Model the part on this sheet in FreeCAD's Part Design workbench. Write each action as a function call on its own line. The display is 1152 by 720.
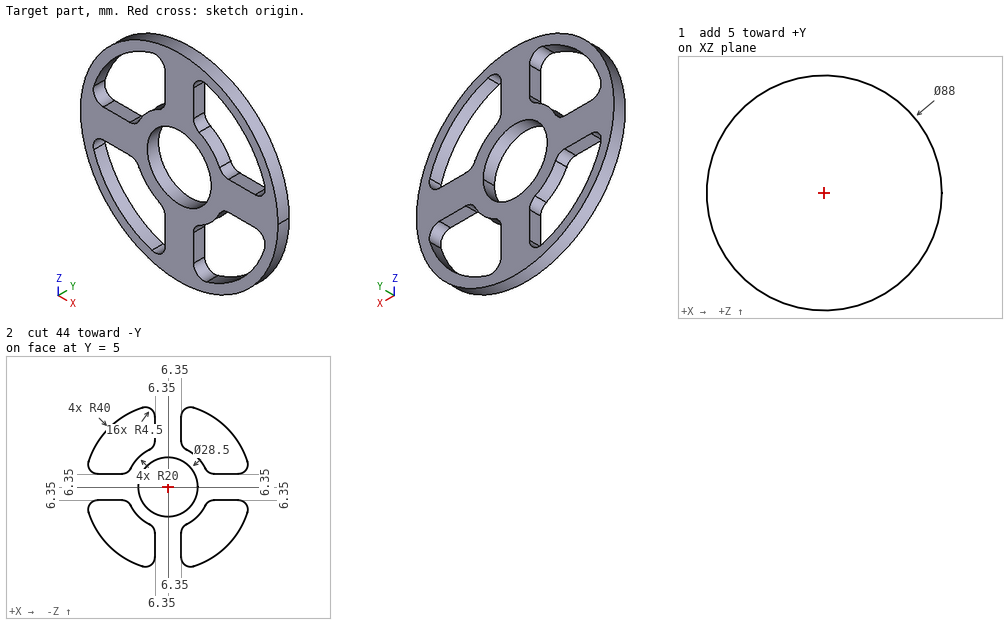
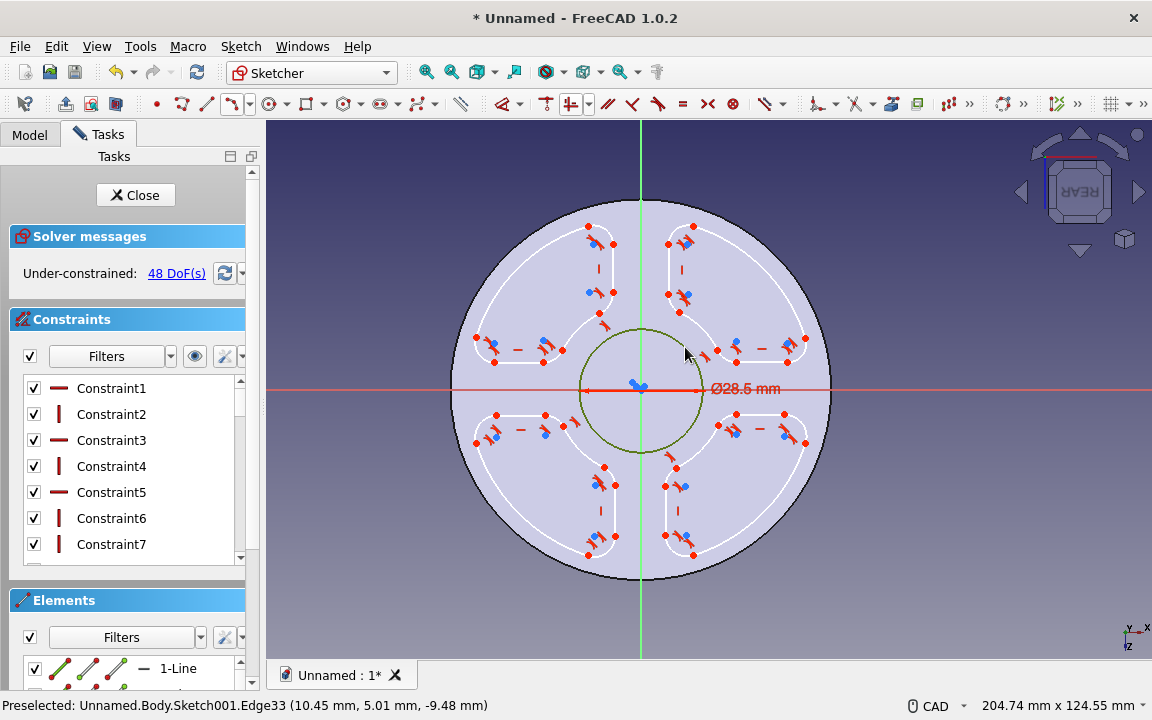
click(586, 322)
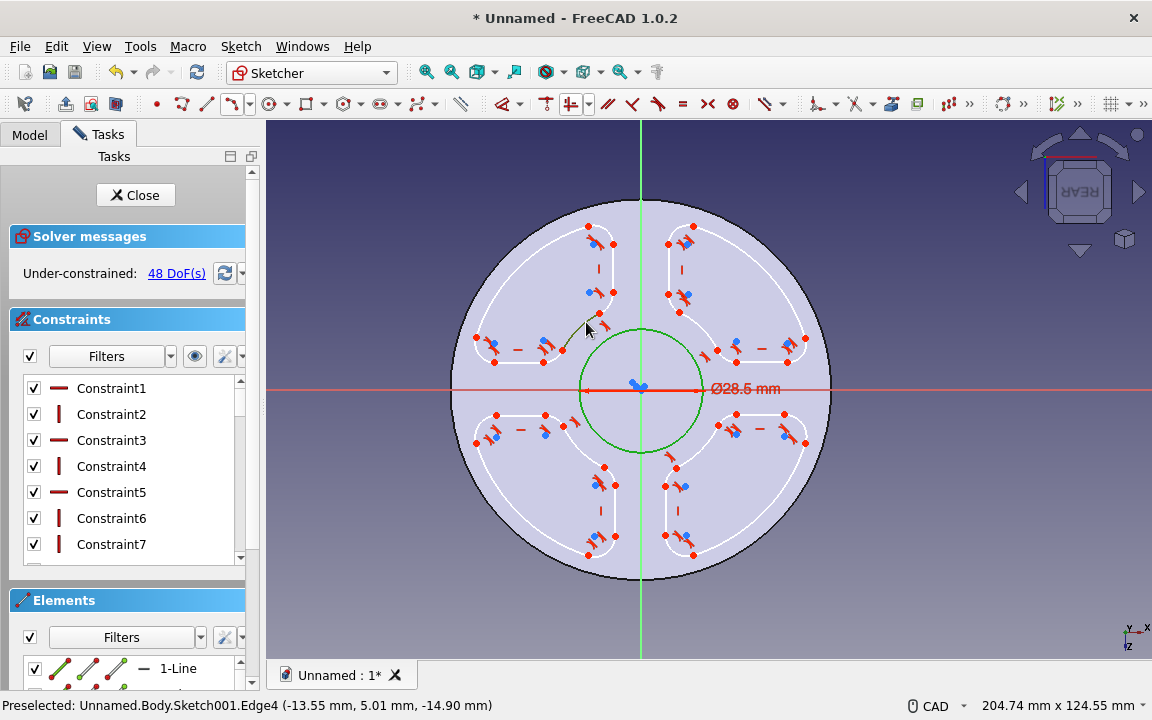
click(546, 104)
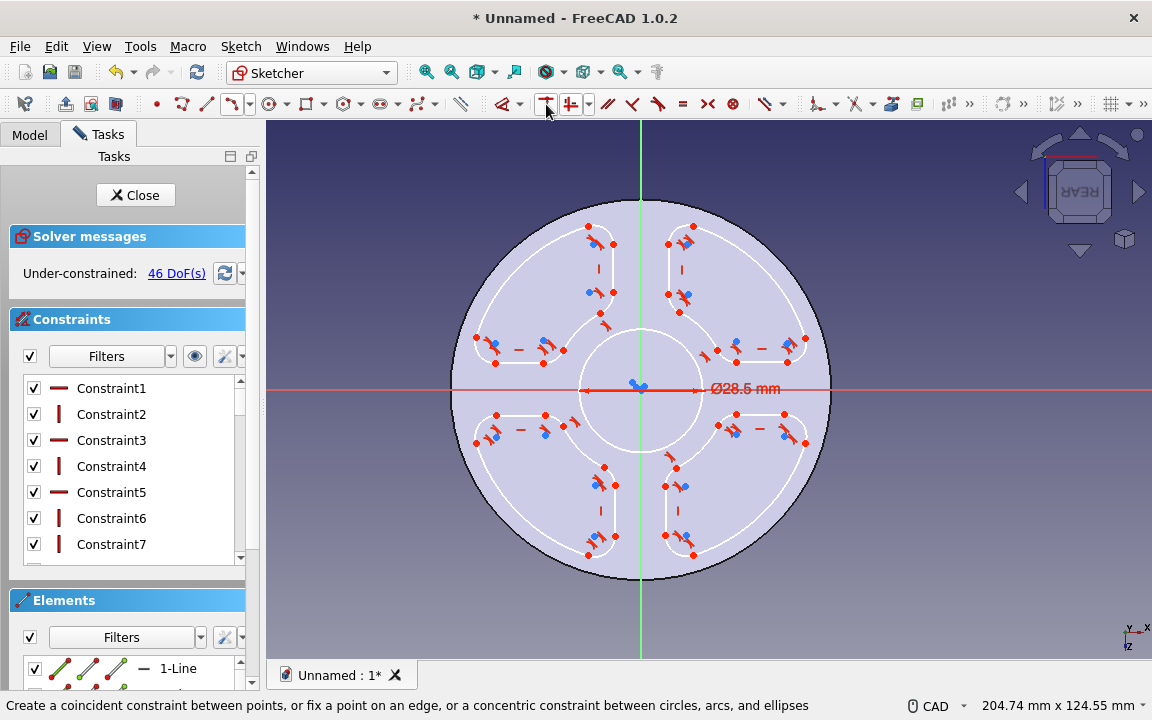
click(685, 347)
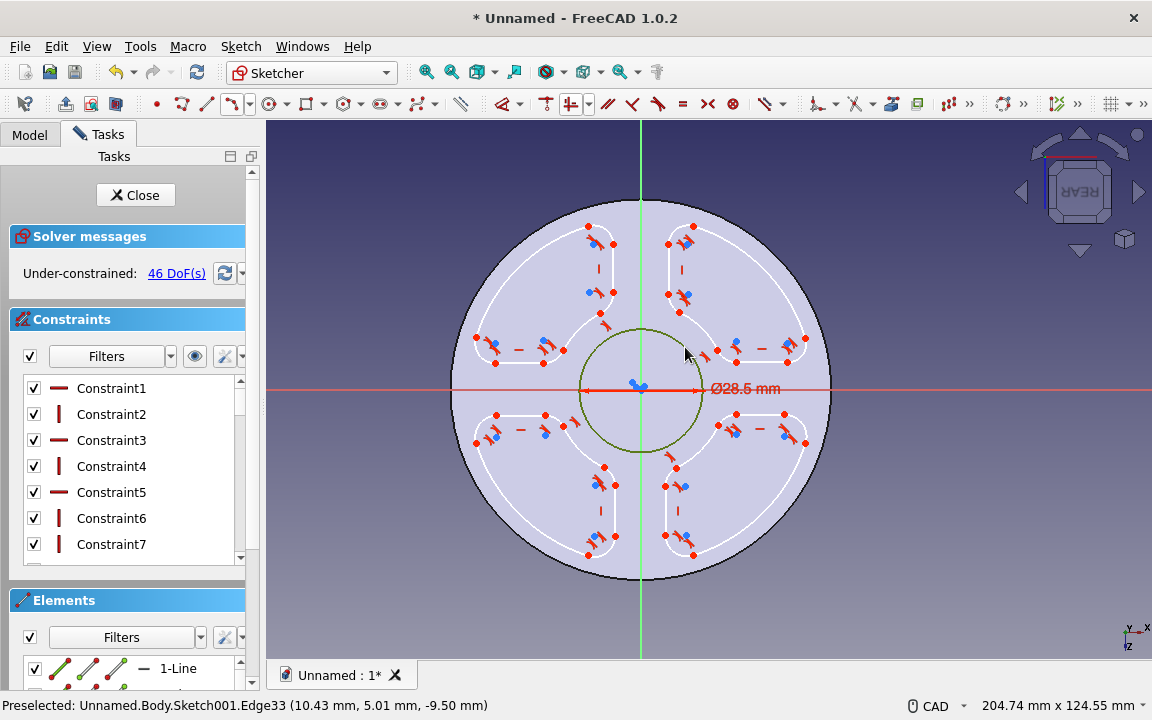
click(544, 247)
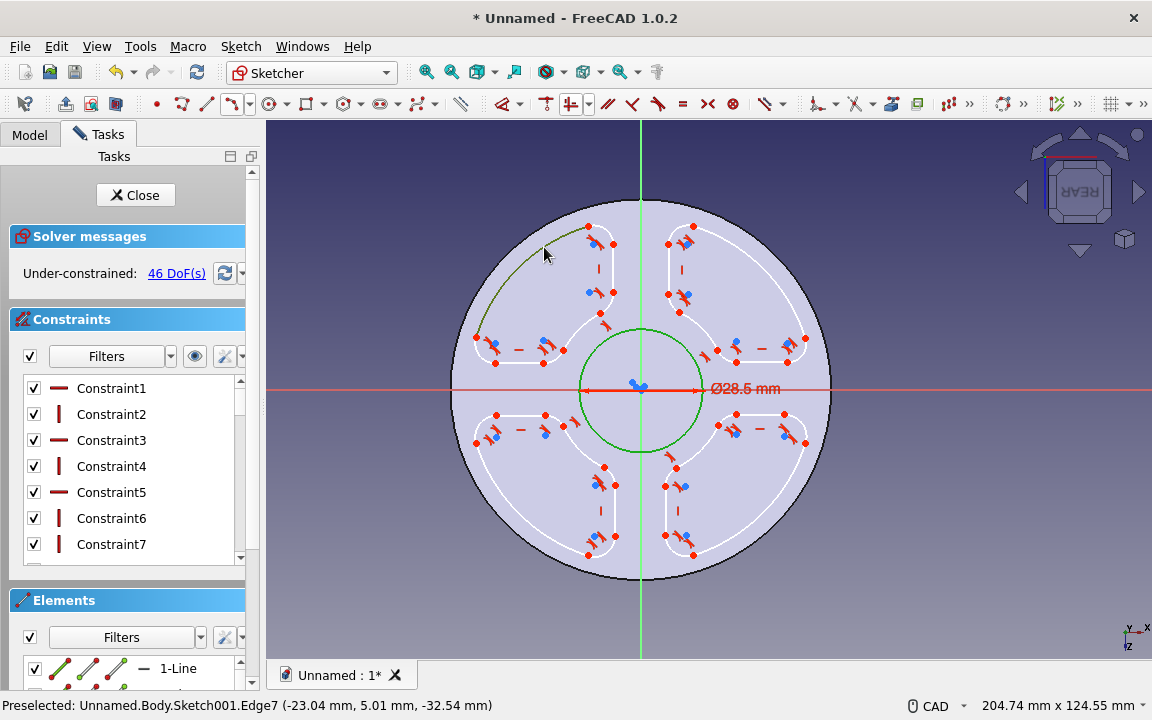
key(c)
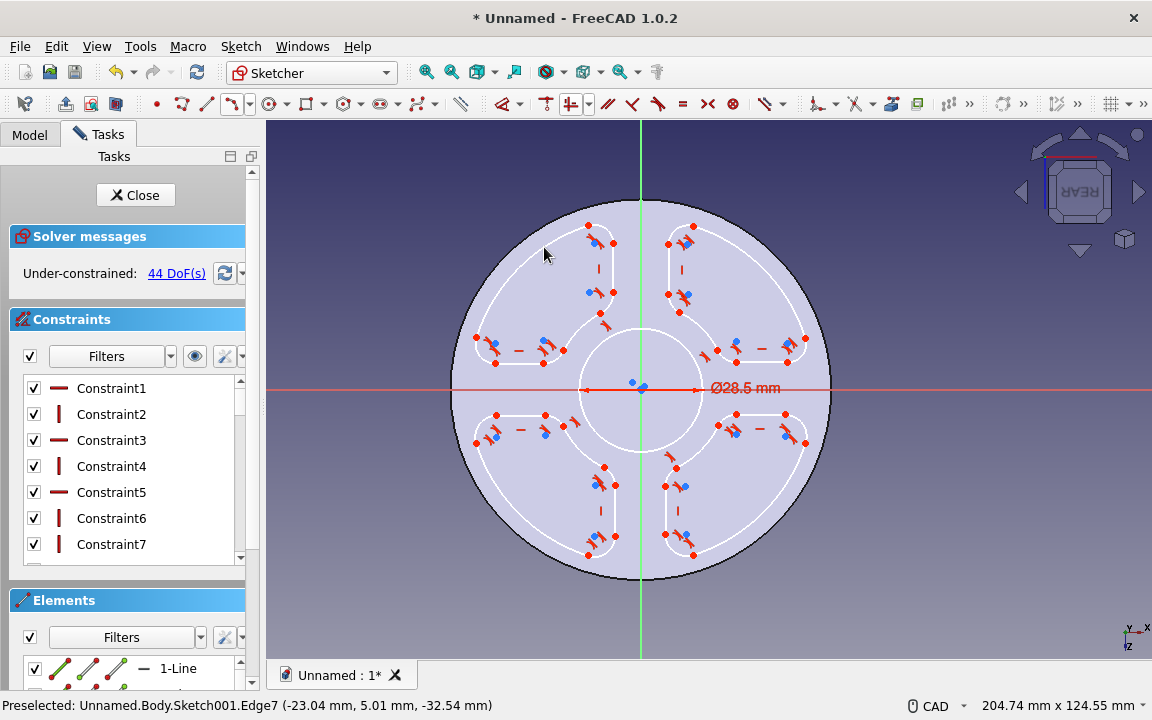
click(684, 347)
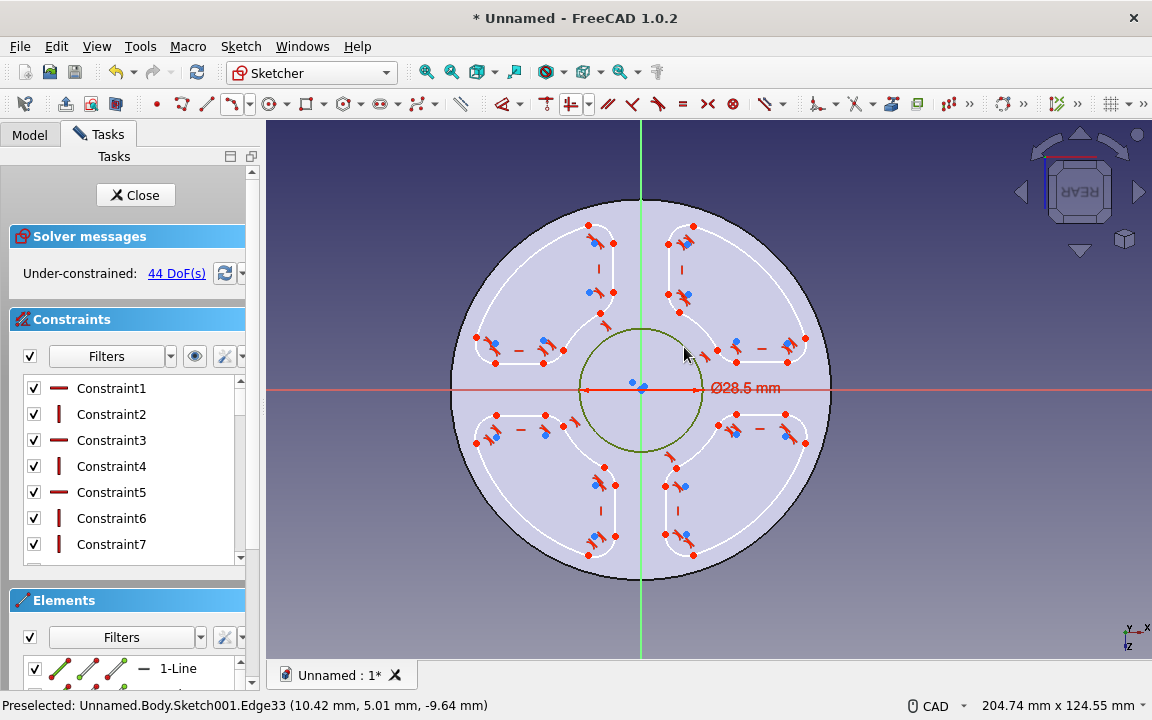
click(784, 294)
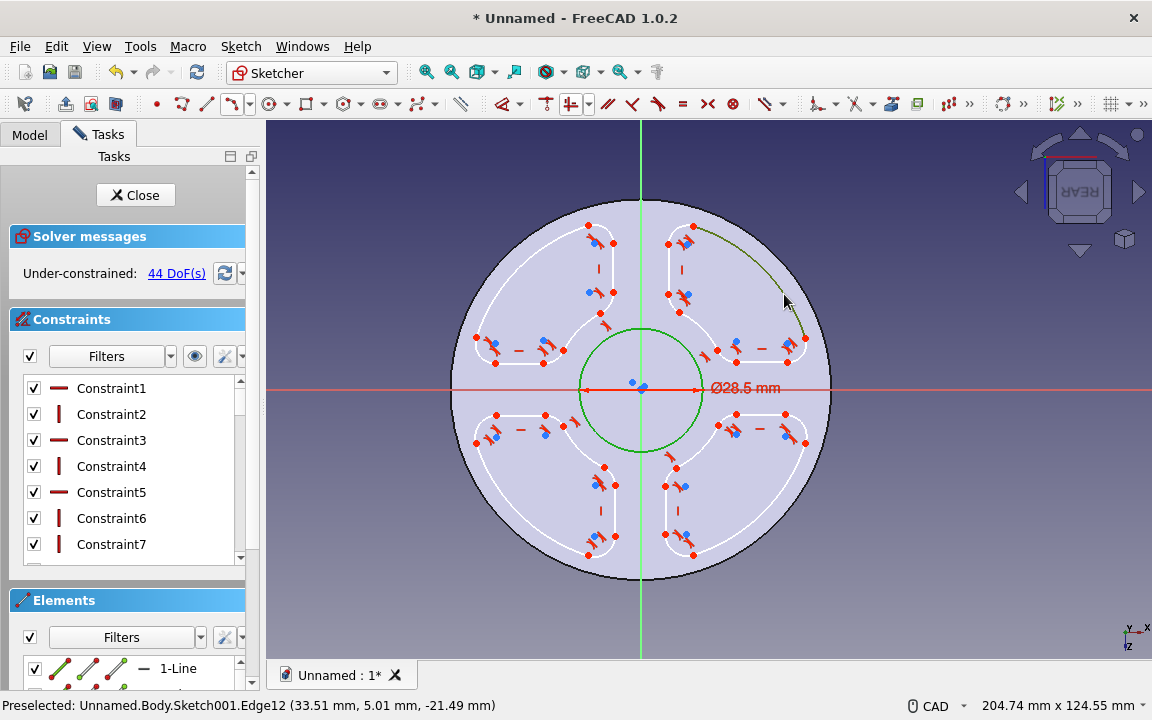
key(c)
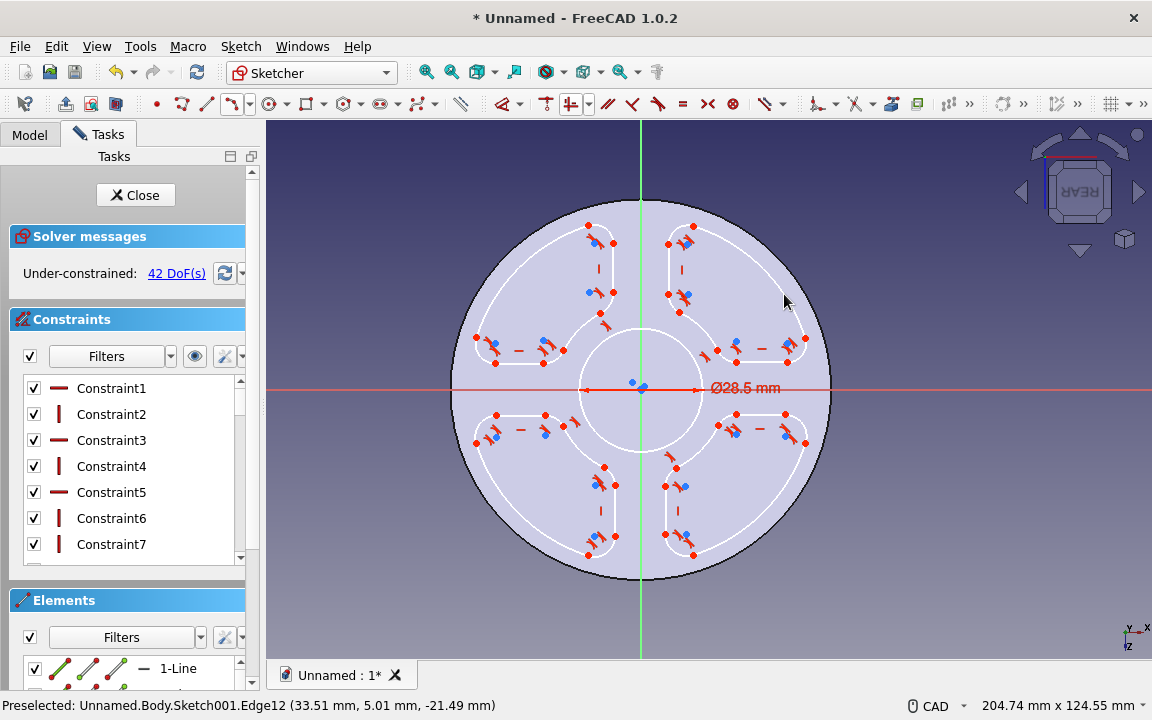
click(684, 347)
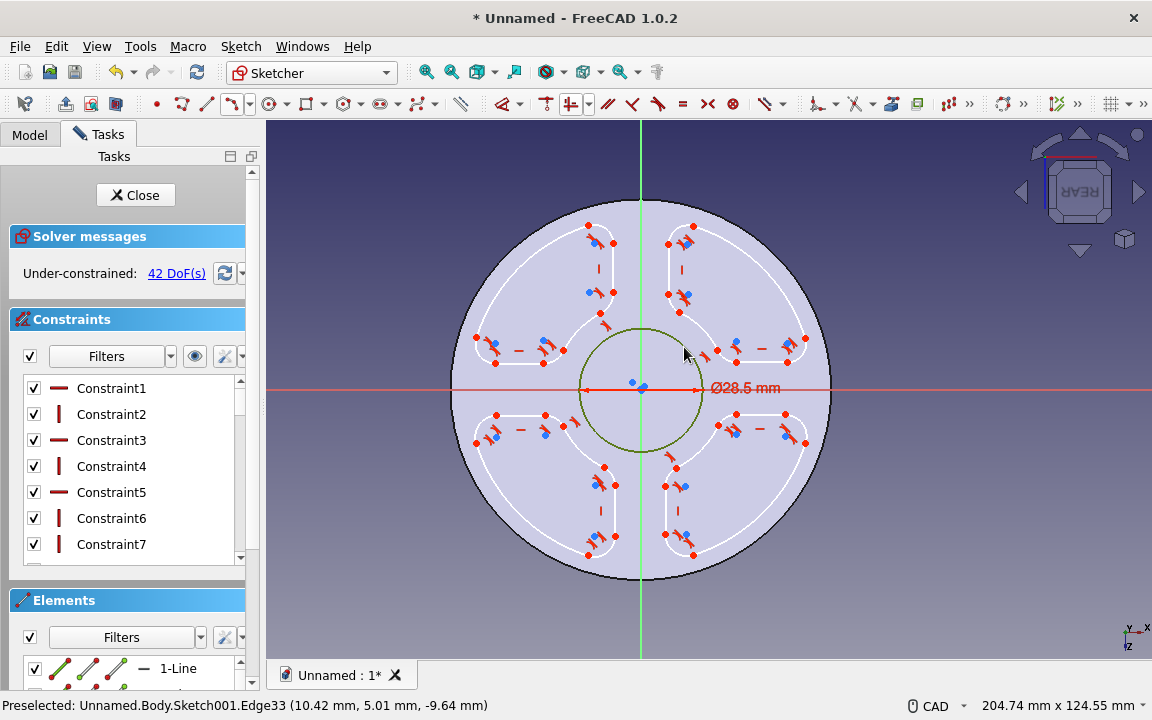
click(709, 337)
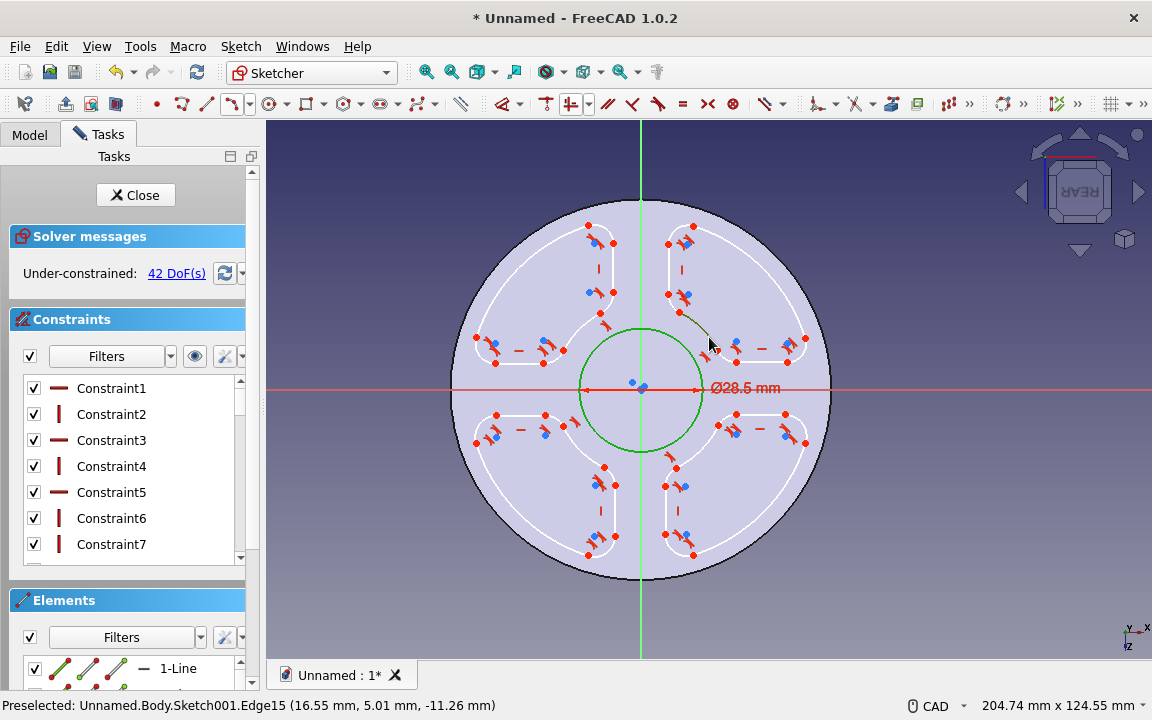
key(c)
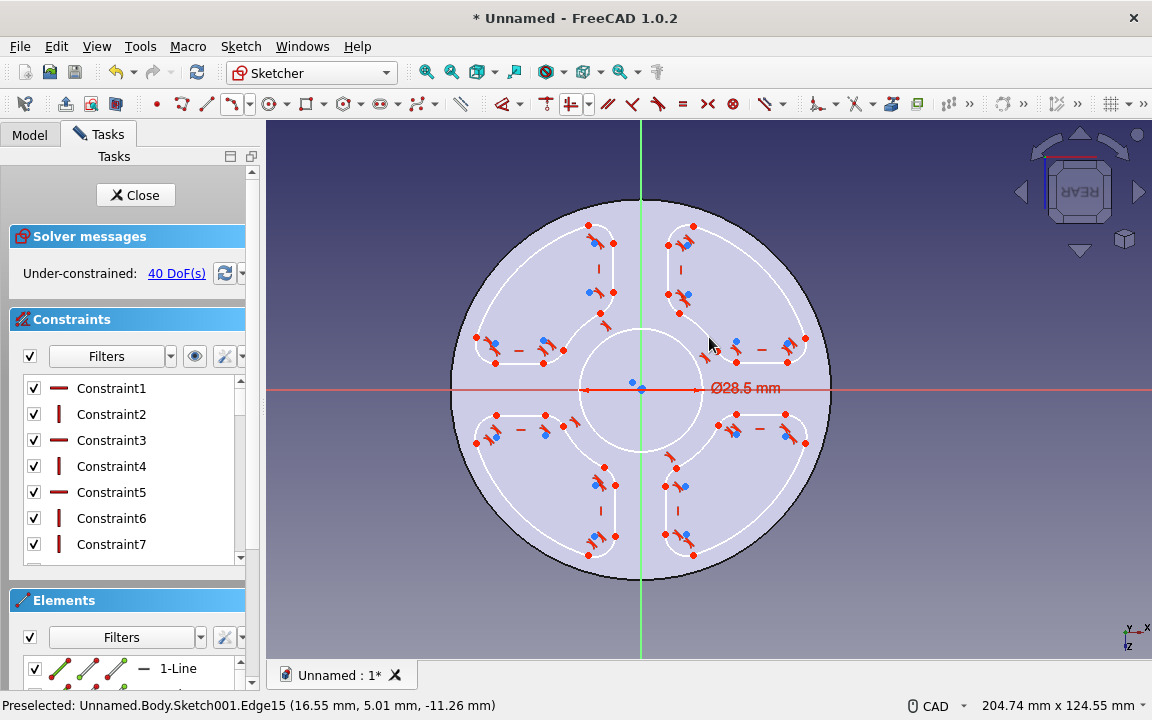
click(685, 347)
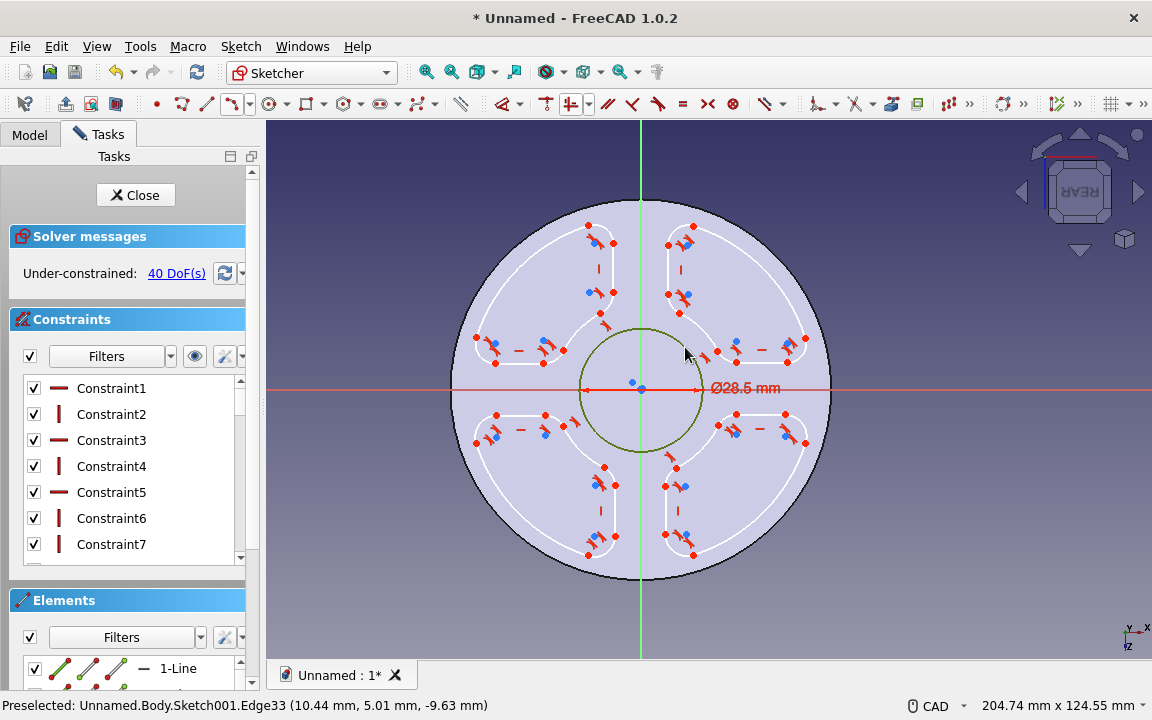
click(692, 458)